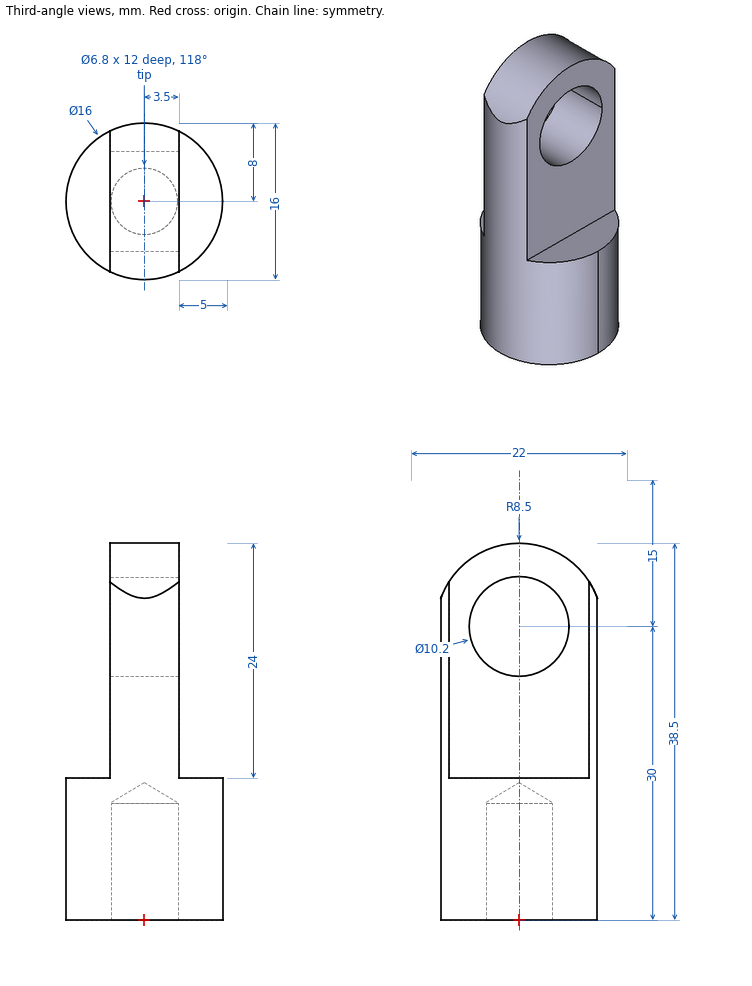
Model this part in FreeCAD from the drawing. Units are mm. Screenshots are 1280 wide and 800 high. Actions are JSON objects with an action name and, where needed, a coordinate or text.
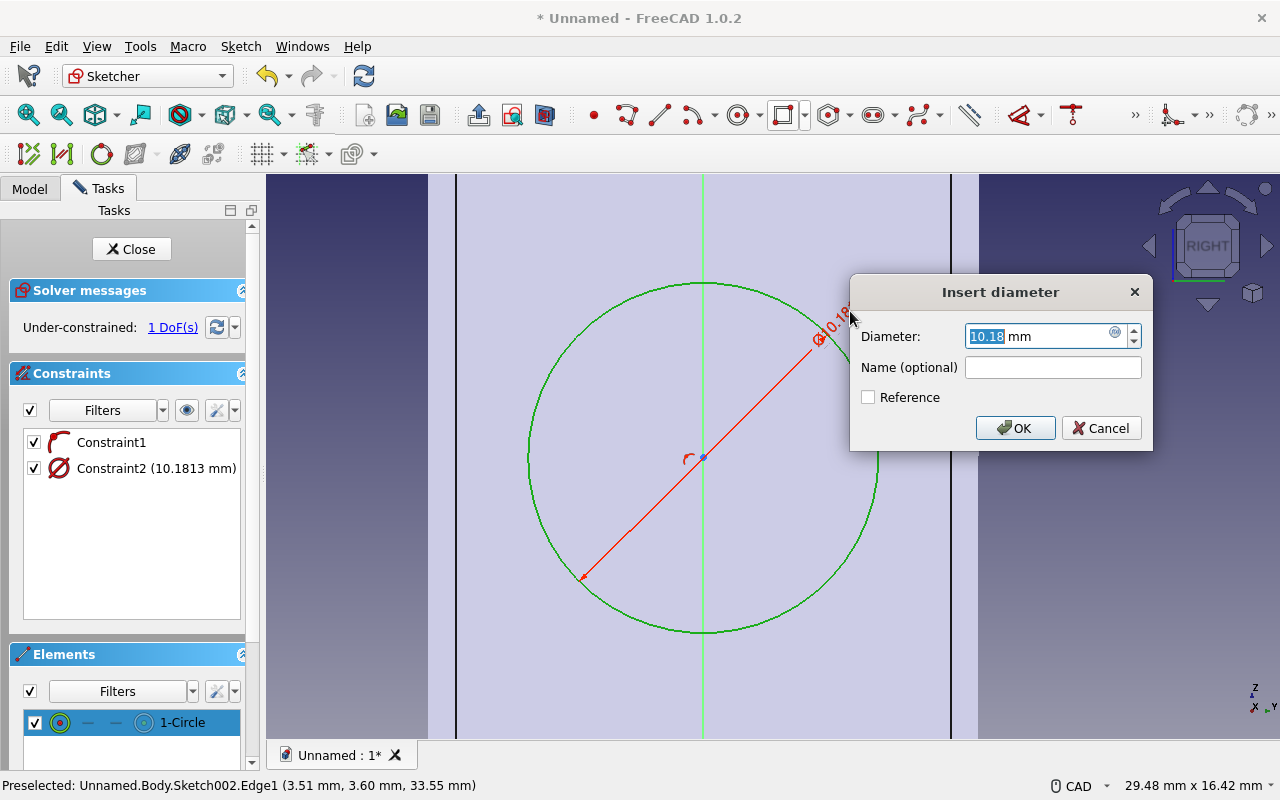
{"action": "type", "text": "10.2"}
{"action": "key", "text": "Return"}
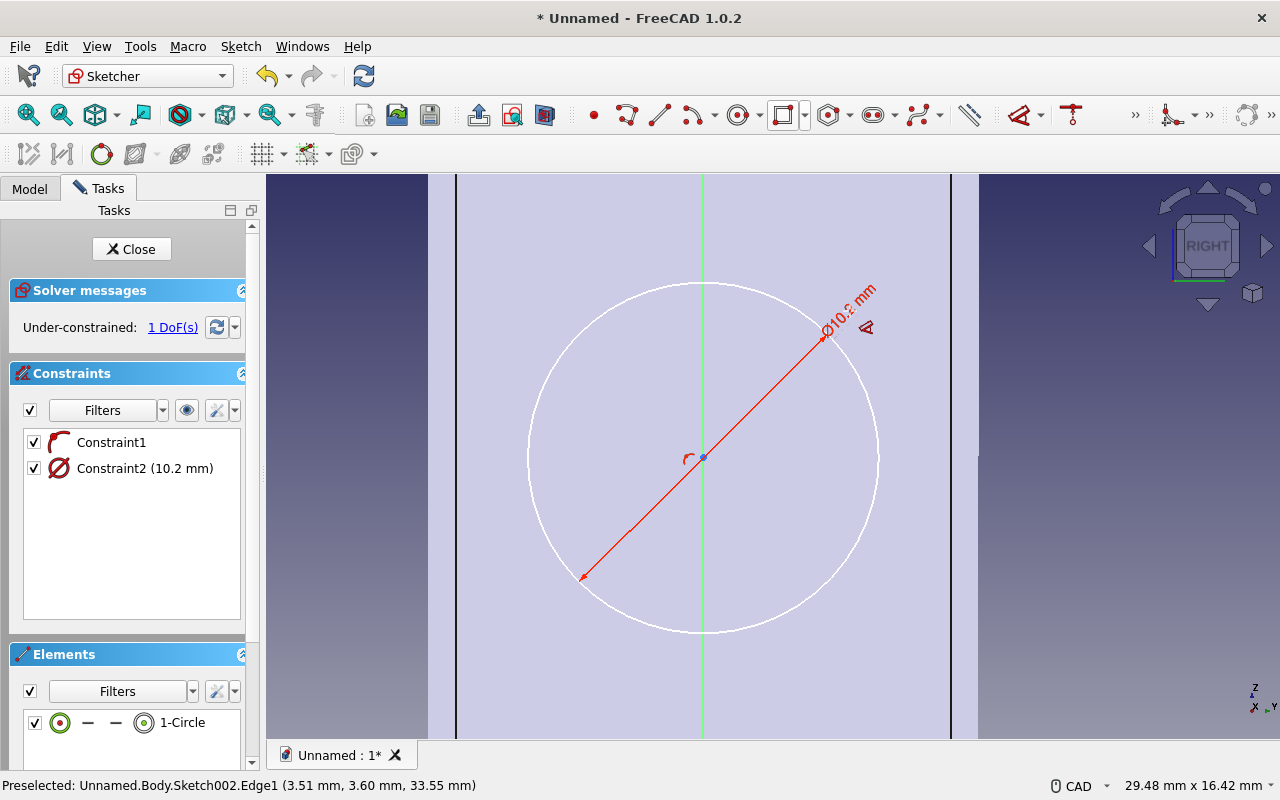
{"action": "left_click", "coordinate": [703, 458]}
{"action": "left_click", "coordinate": [737, 585]}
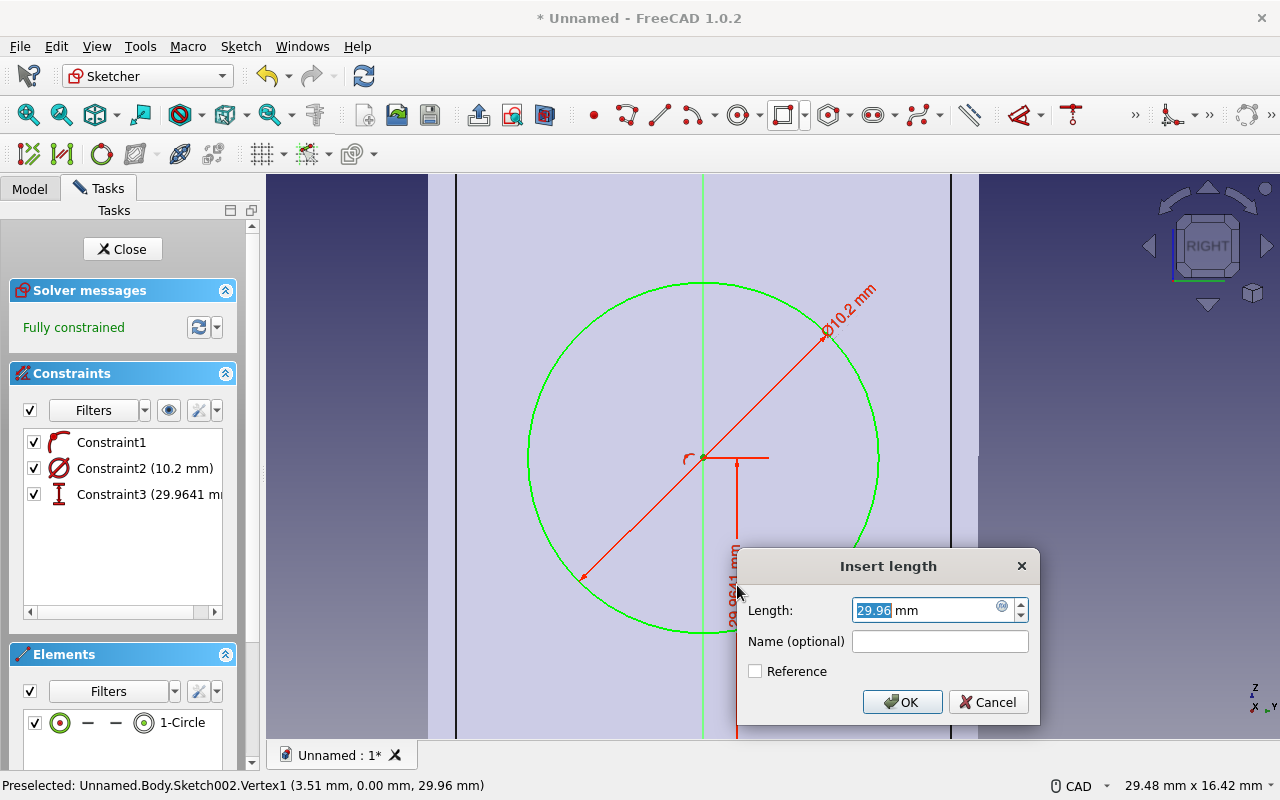
{"action": "type", "text": "30"}
{"action": "key", "text": "Return"}
{"action": "key", "text": "Escape"}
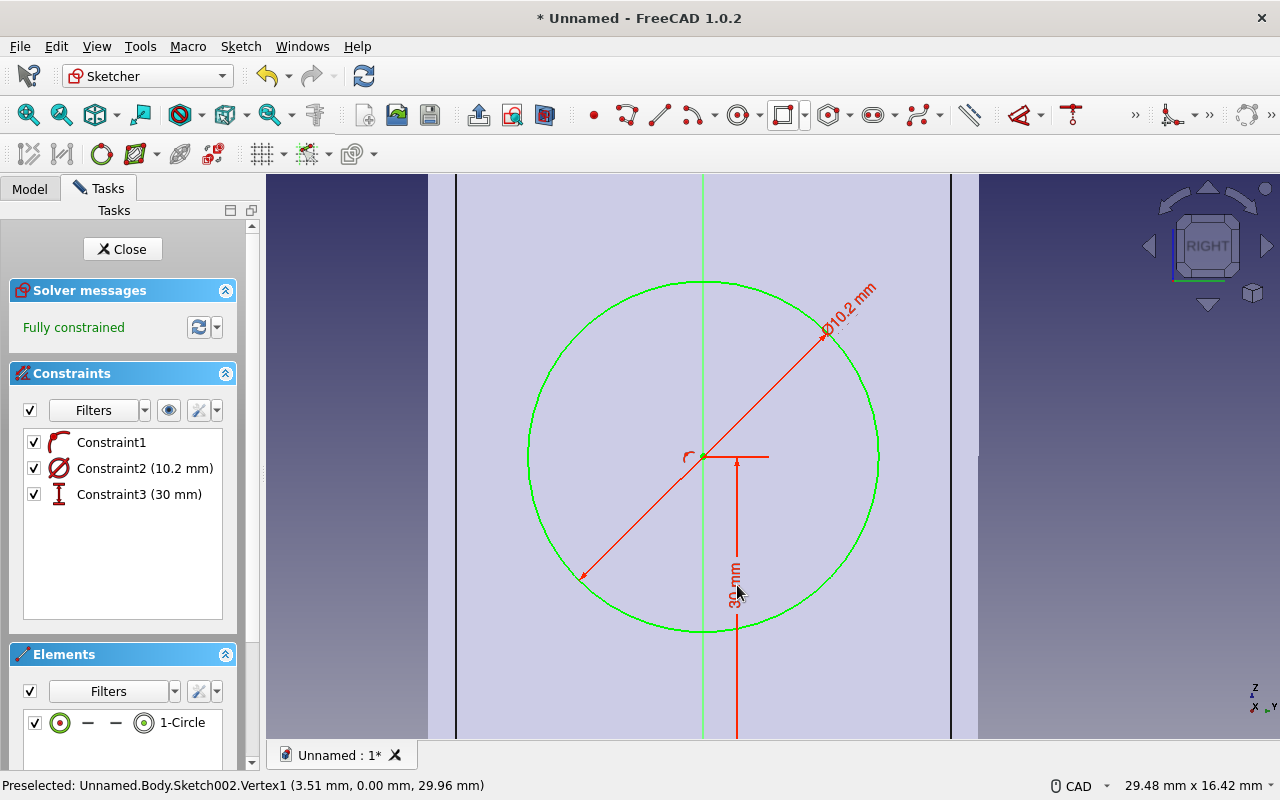
{"action": "left_click", "coordinate": [123, 249]}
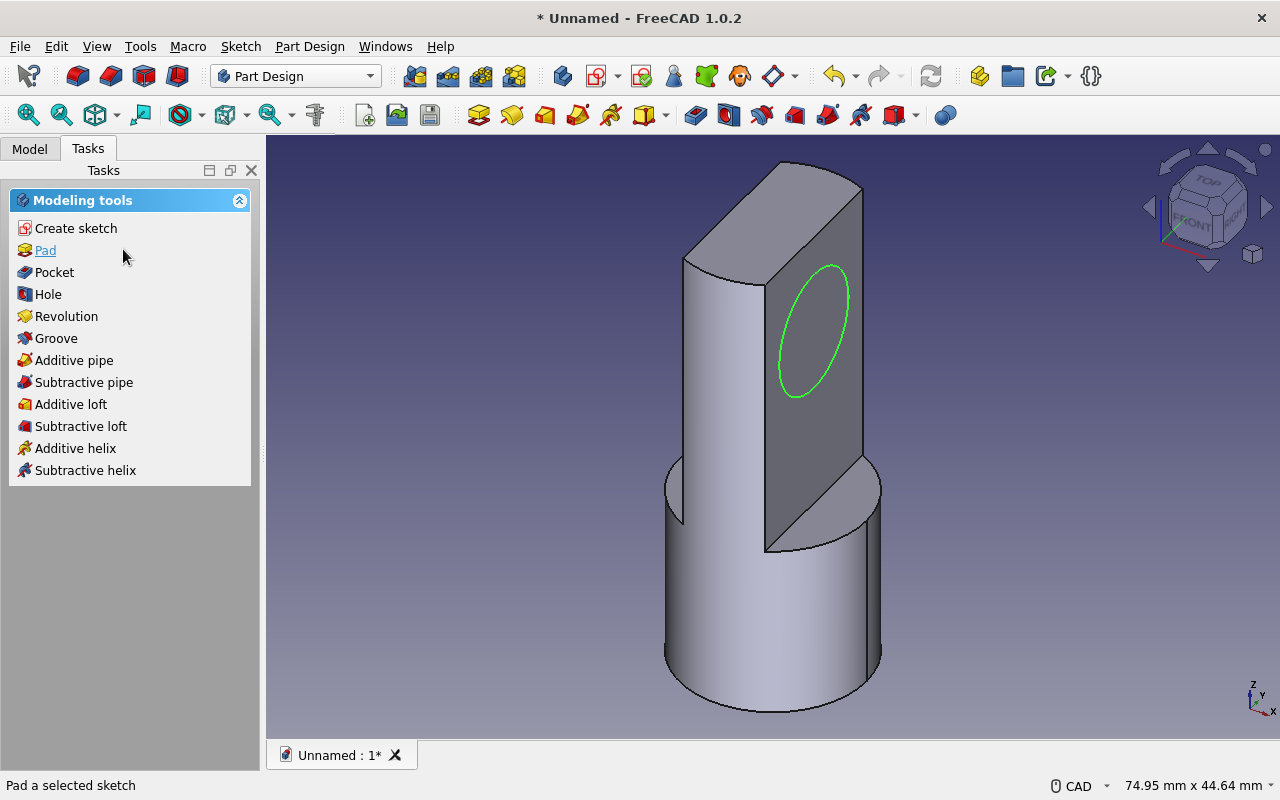
{"action": "left_click", "coordinate": [696, 116]}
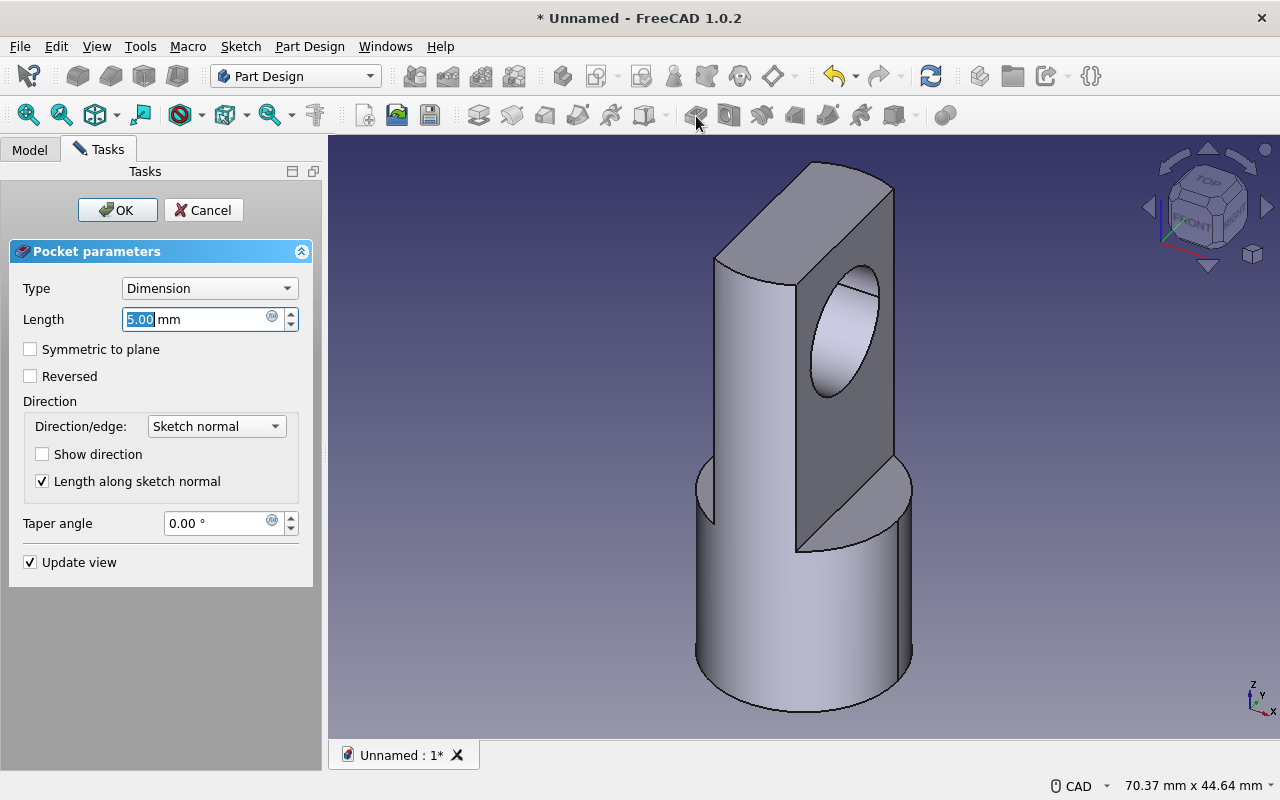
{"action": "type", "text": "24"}
{"action": "key", "text": "Tab"}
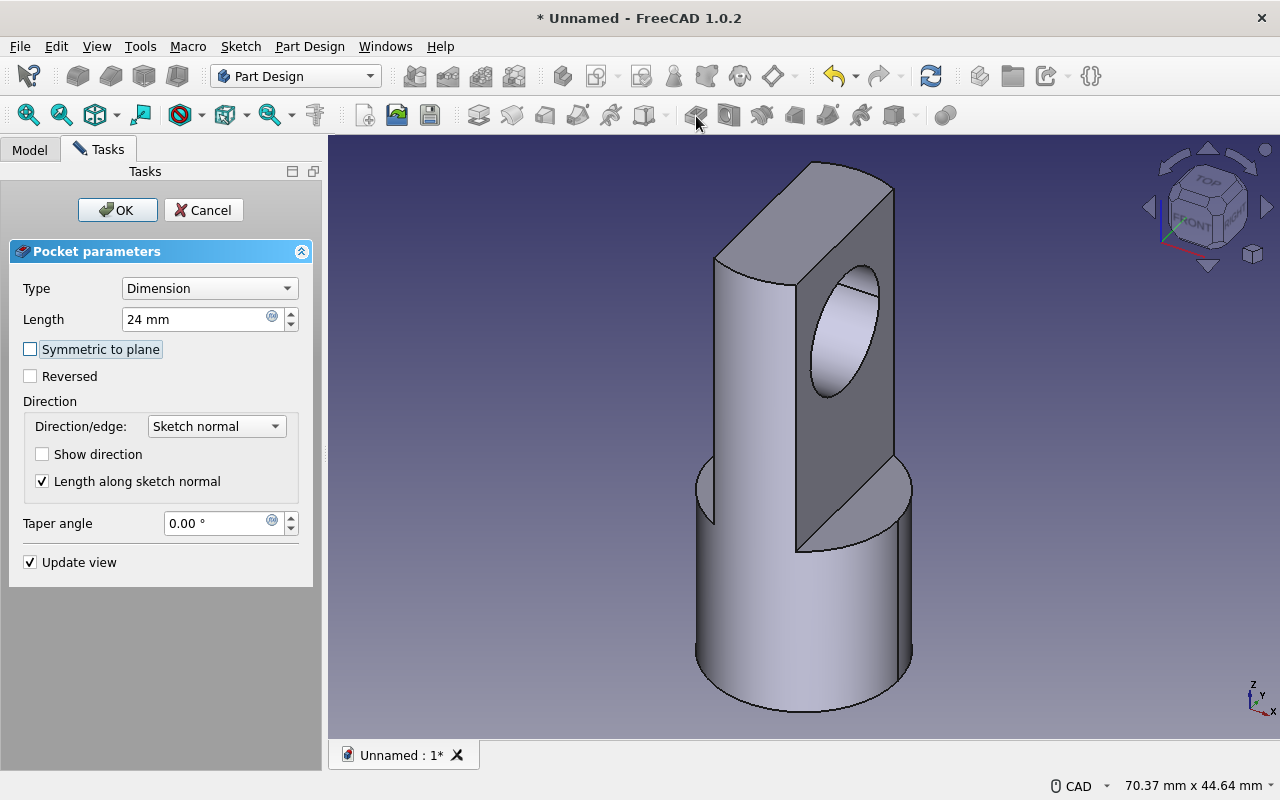
{"action": "left_click", "coordinate": [118, 210]}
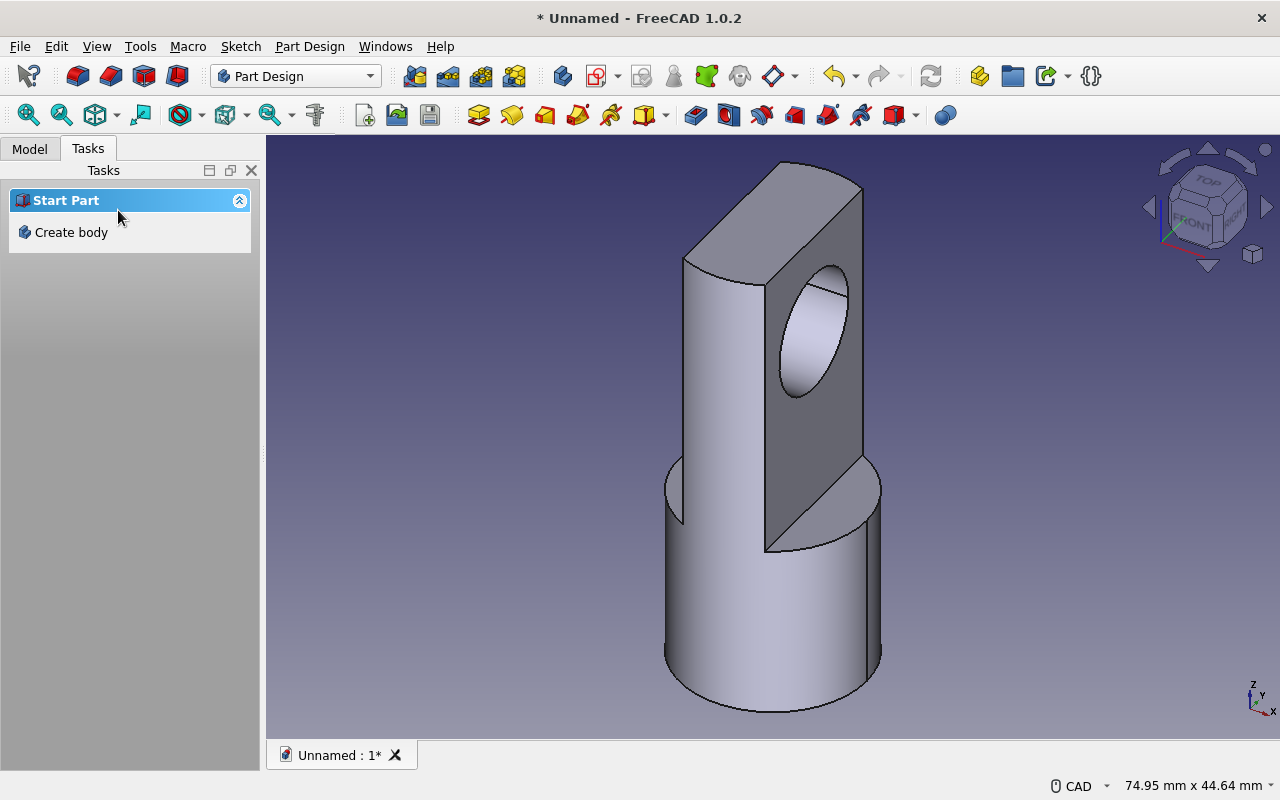
{"action": "left_click", "coordinate": [814, 445]}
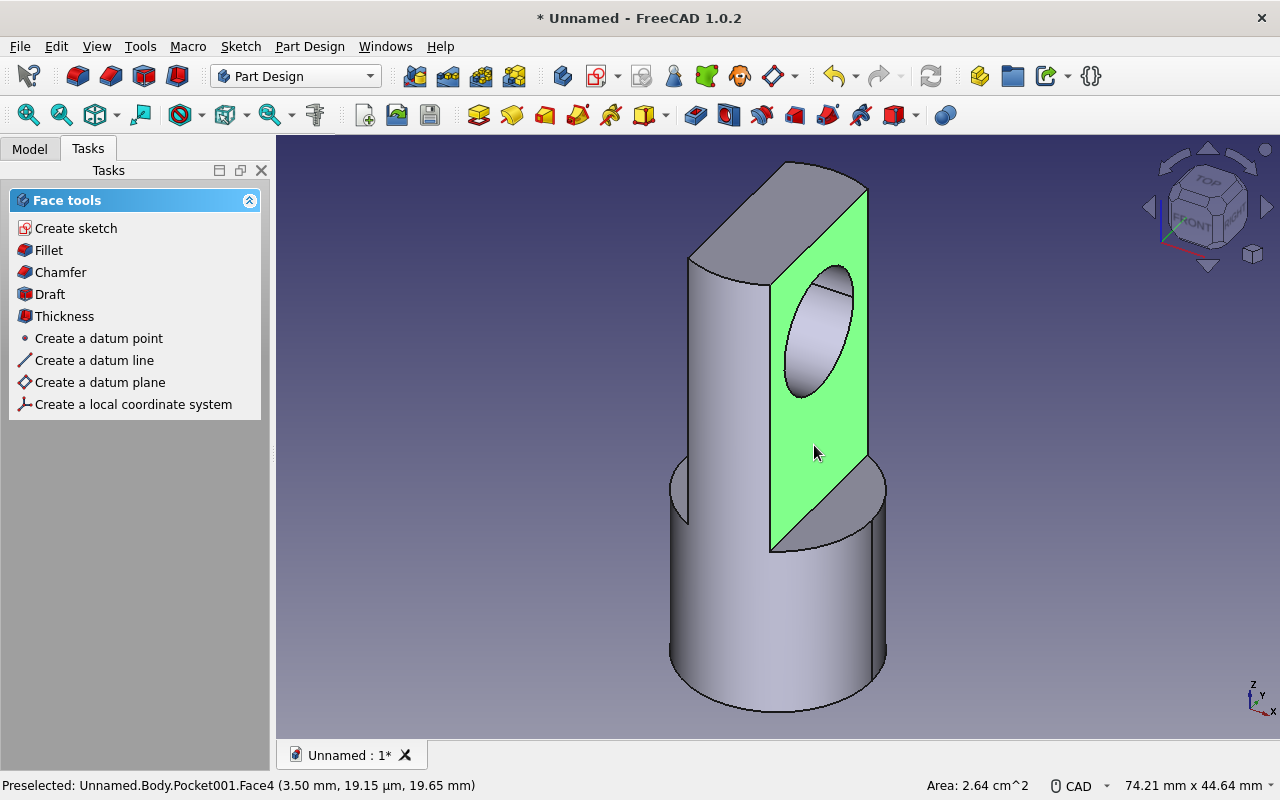
{"action": "left_click", "coordinate": [596, 76]}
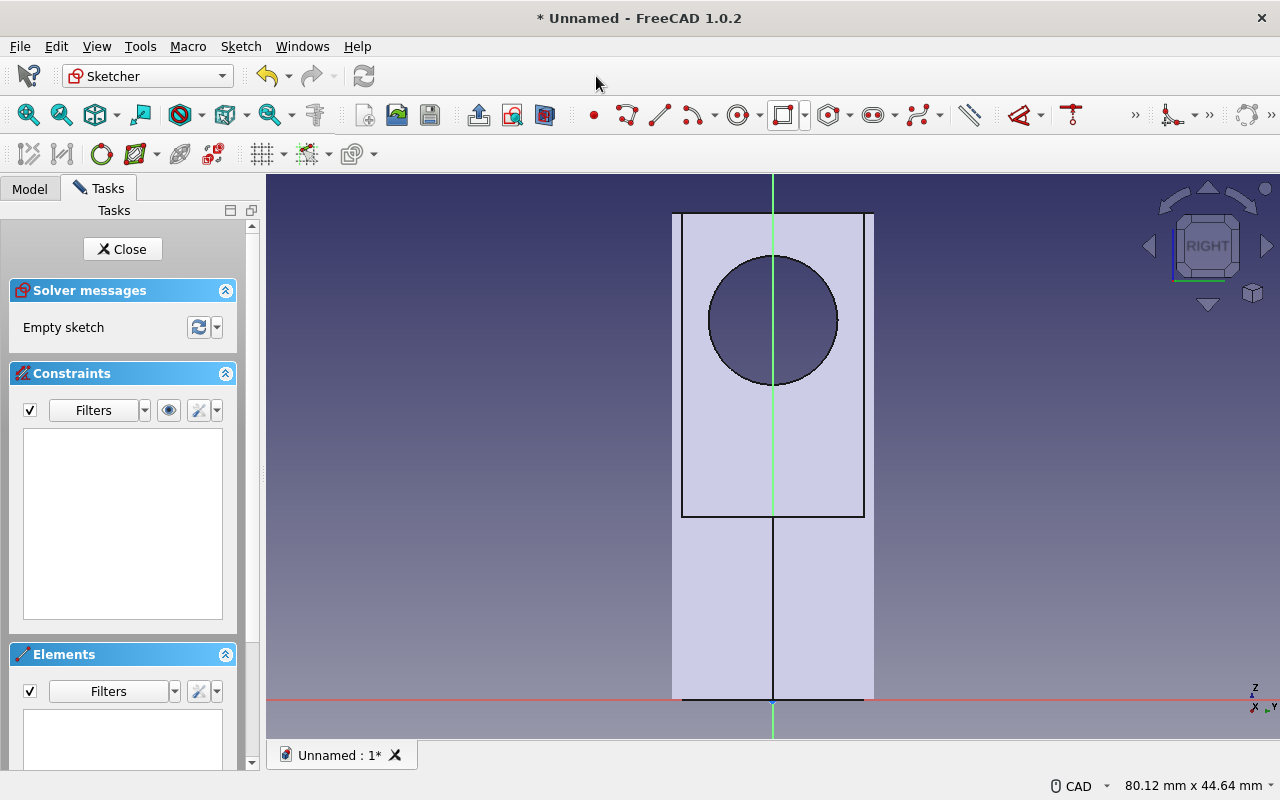
{"action": "left_click", "coordinate": [545, 116]}